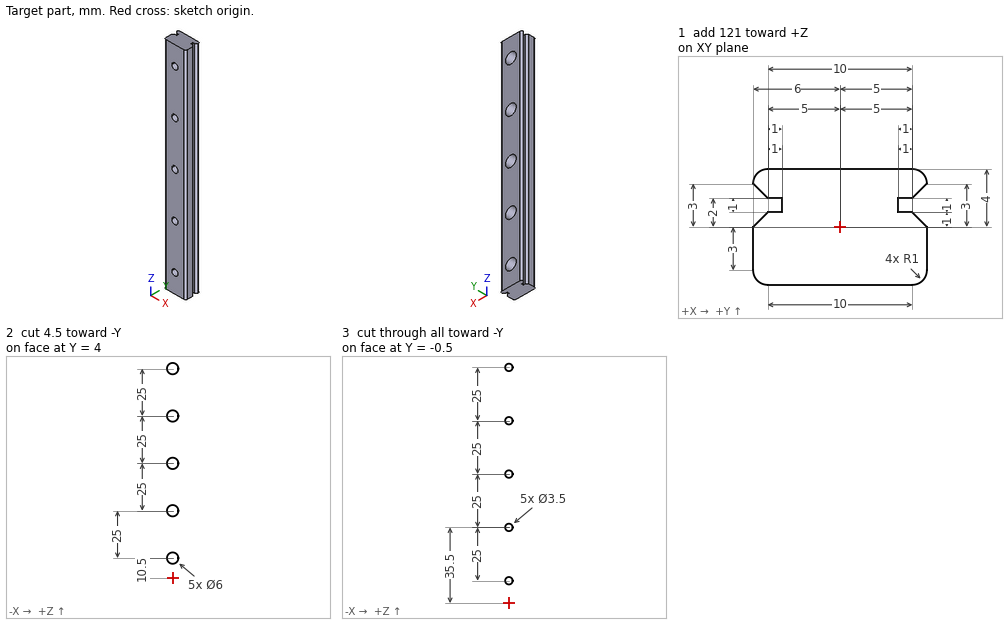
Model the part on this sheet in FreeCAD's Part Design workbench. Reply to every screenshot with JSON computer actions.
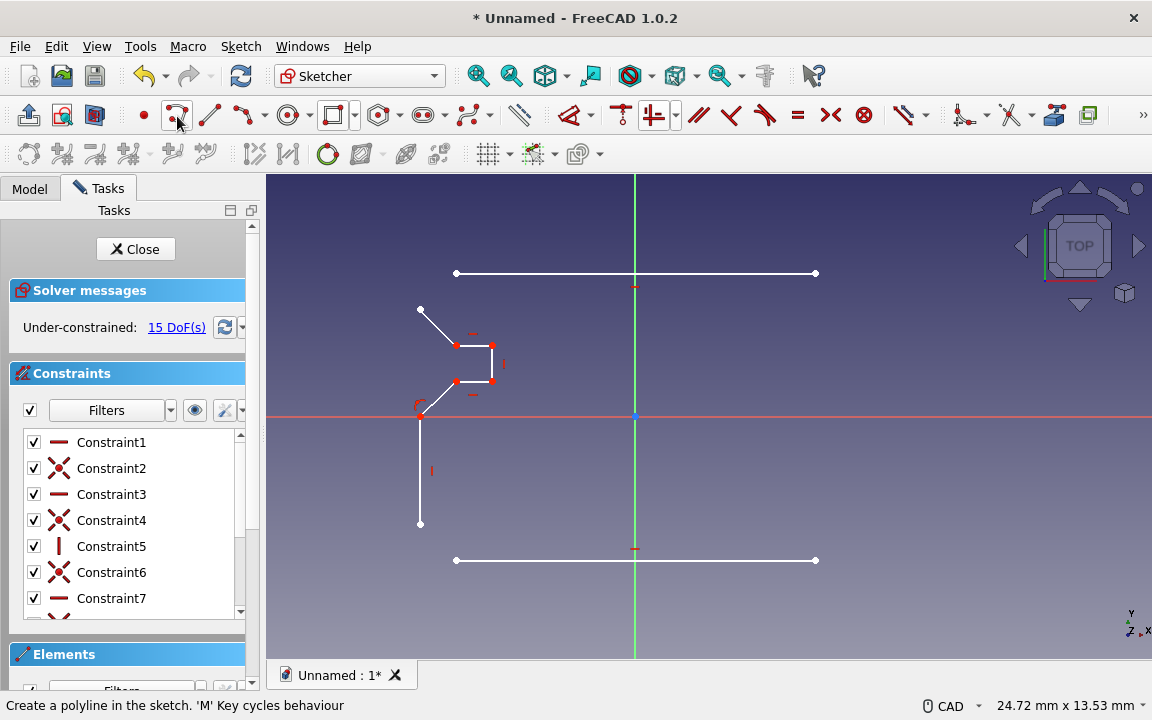
{"action": "left_click", "coordinate": [850, 524]}
{"action": "left_click", "coordinate": [850, 416]}
{"action": "left_click", "coordinate": [815, 381]}
{"action": "left_click", "coordinate": [779, 381]}
{"action": "left_click", "coordinate": [779, 345]}
{"action": "left_click", "coordinate": [815, 345]}
{"action": "left_click", "coordinate": [850, 309]}
{"action": "right_click", "coordinate": [850, 309]}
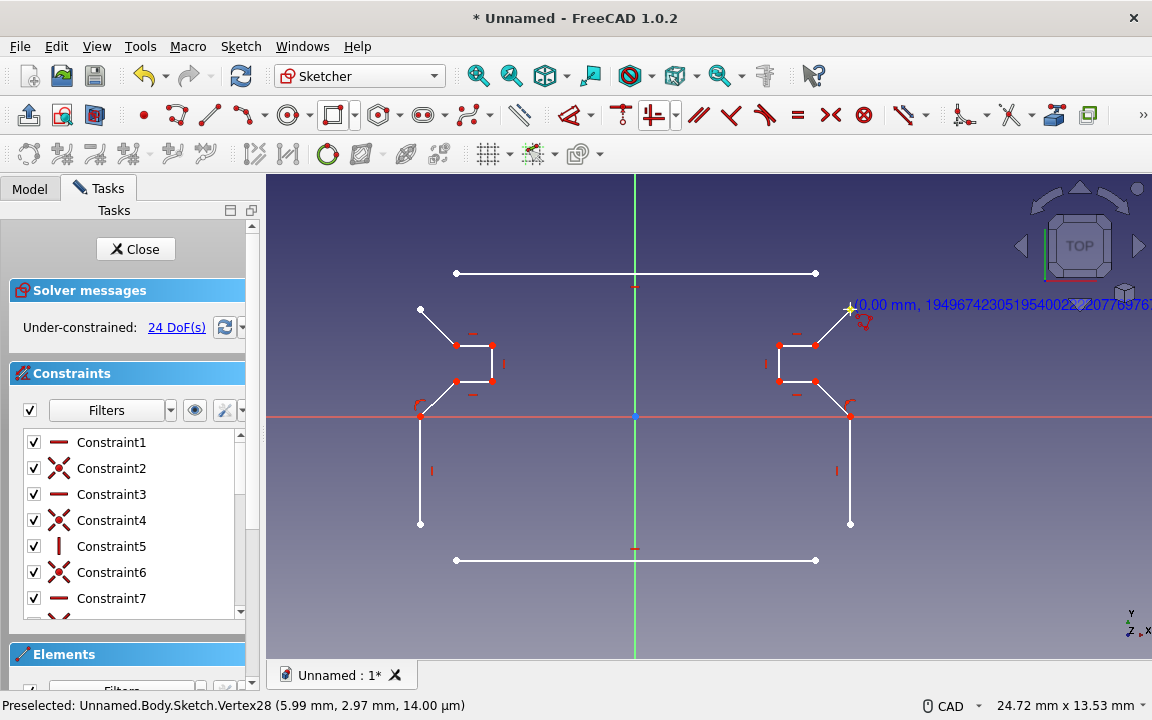
{"action": "left_click", "coordinate": [242, 116]}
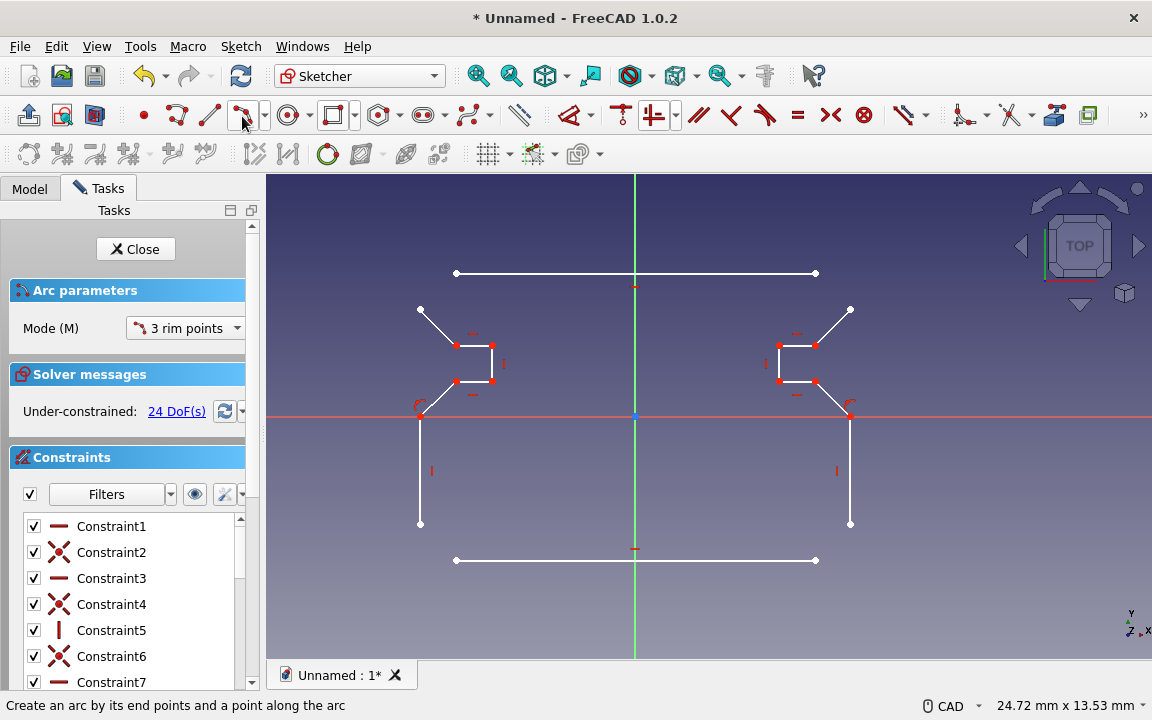
{"action": "left_click", "coordinate": [456, 274]}
{"action": "left_click", "coordinate": [420, 310]}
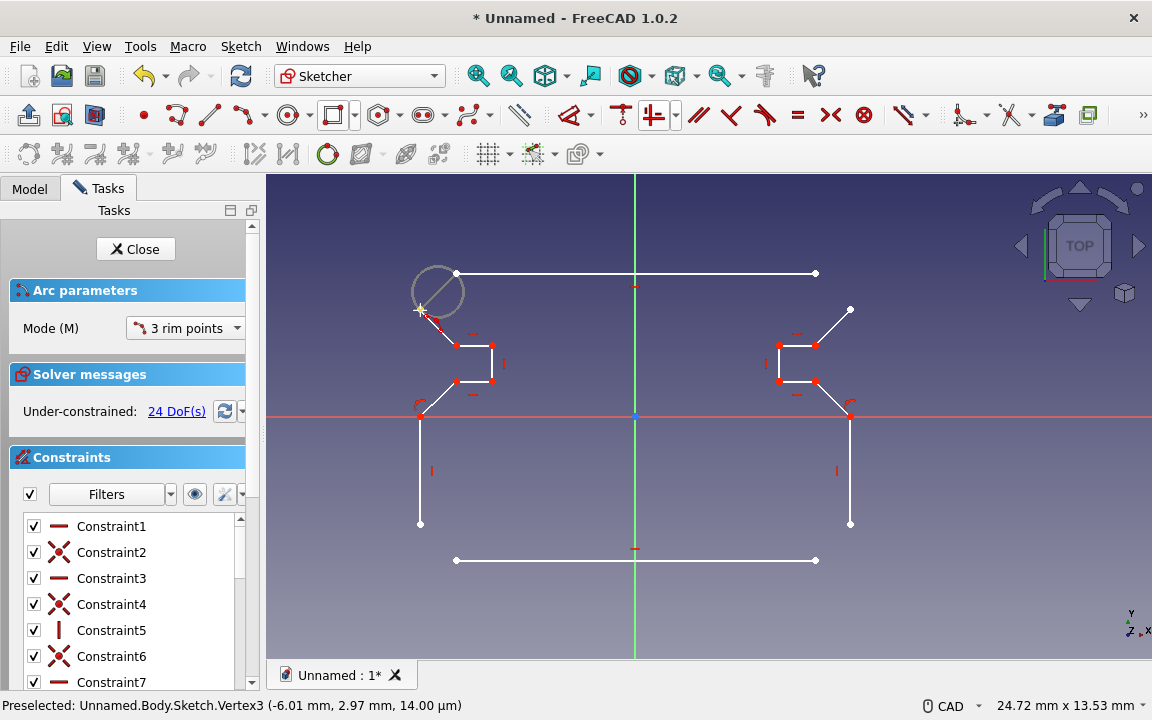
{"action": "scroll", "coordinate": [431, 284], "scroll_direction": "up", "scroll_amount": 3}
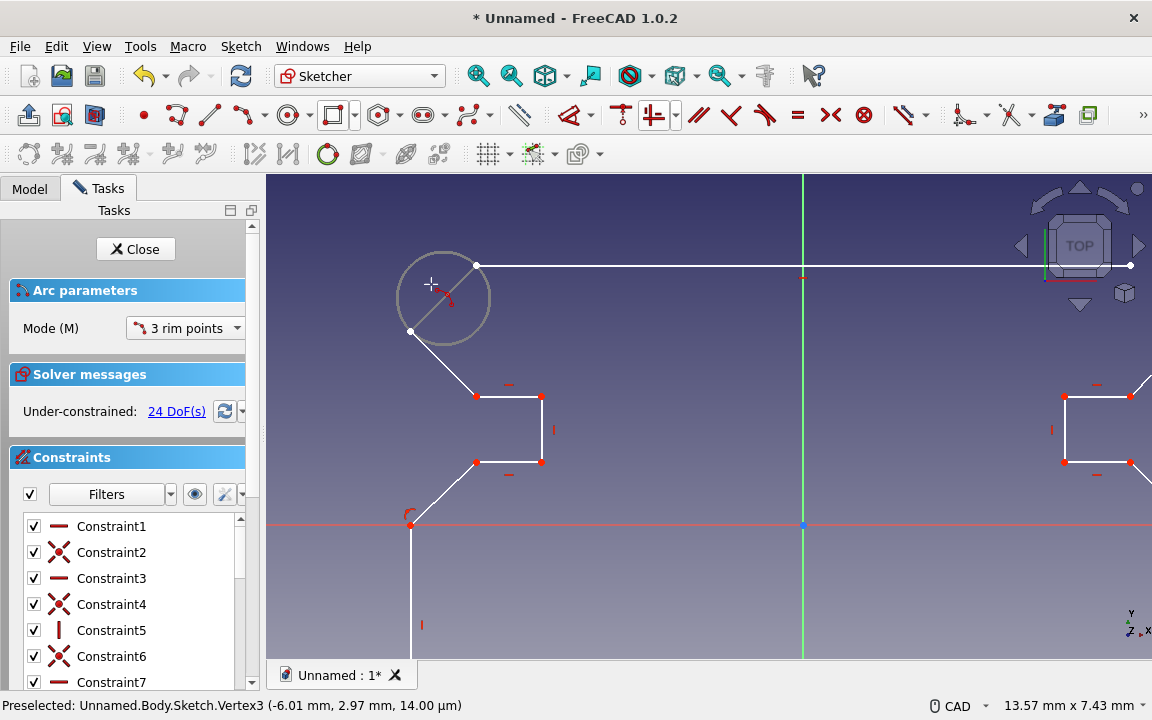
{"action": "left_click", "coordinate": [431, 283]}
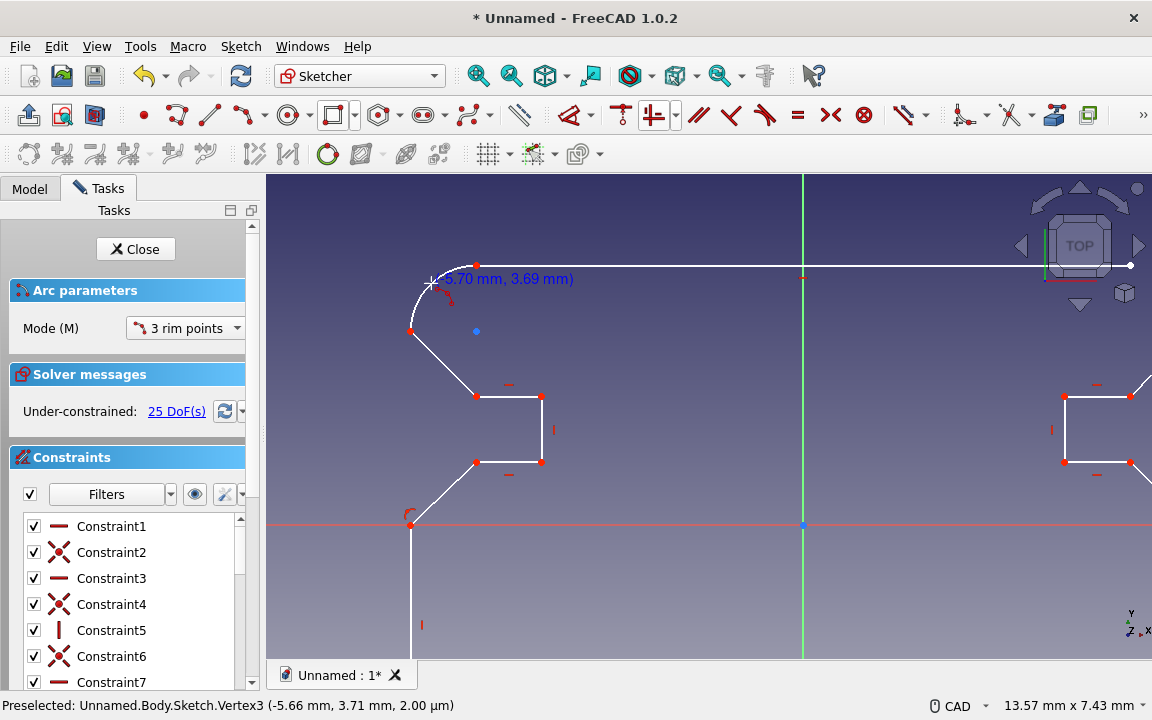
{"action": "scroll", "coordinate": [442, 284], "scroll_direction": "down", "scroll_amount": 3}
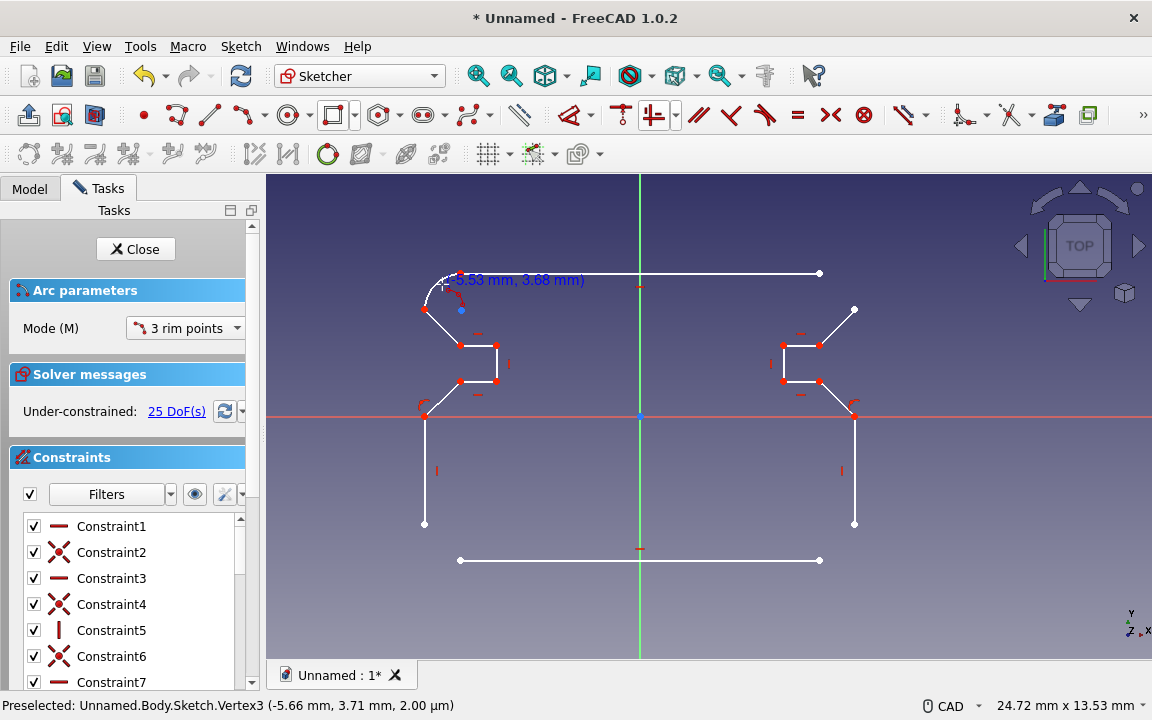
{"action": "left_click", "coordinate": [425, 525]}
{"action": "left_click", "coordinate": [461, 561]}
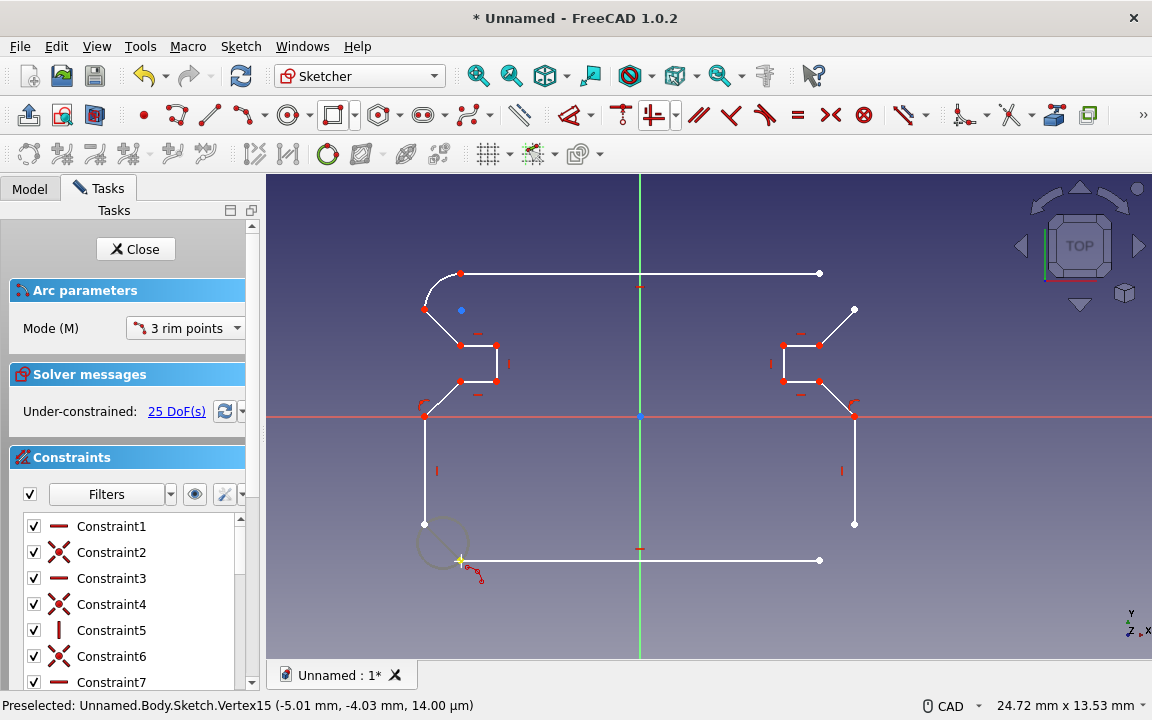
{"action": "scroll", "coordinate": [436, 549], "scroll_direction": "up", "scroll_amount": 3}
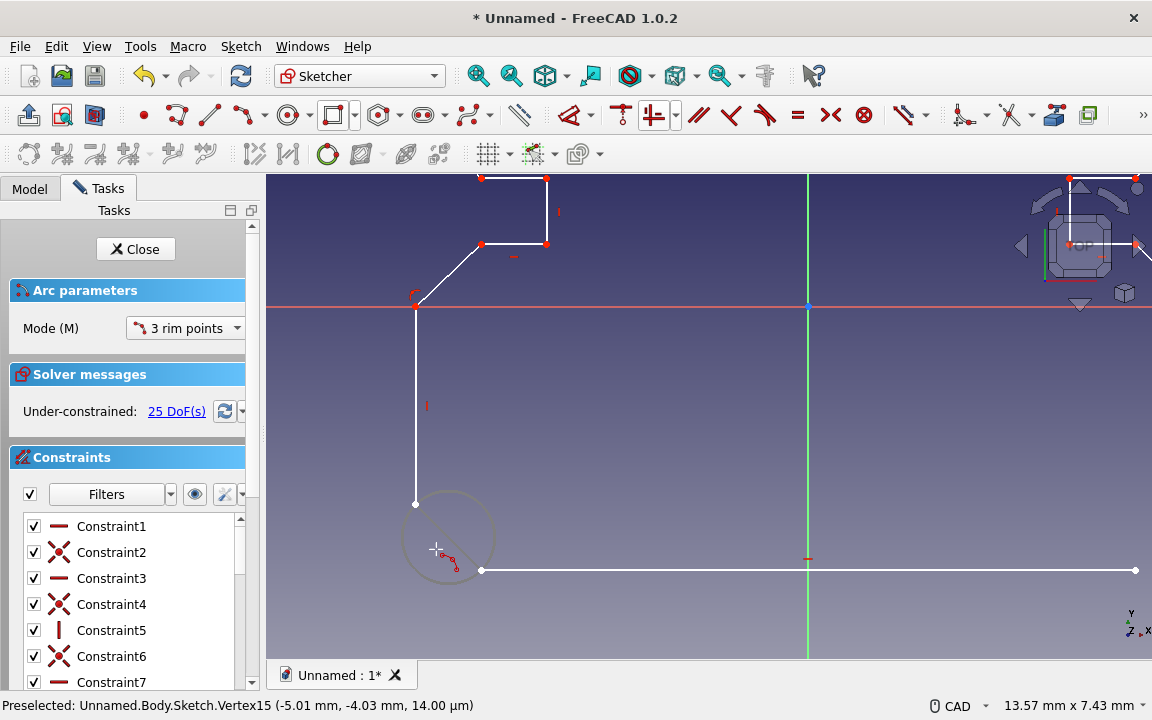
{"action": "left_click", "coordinate": [436, 549]}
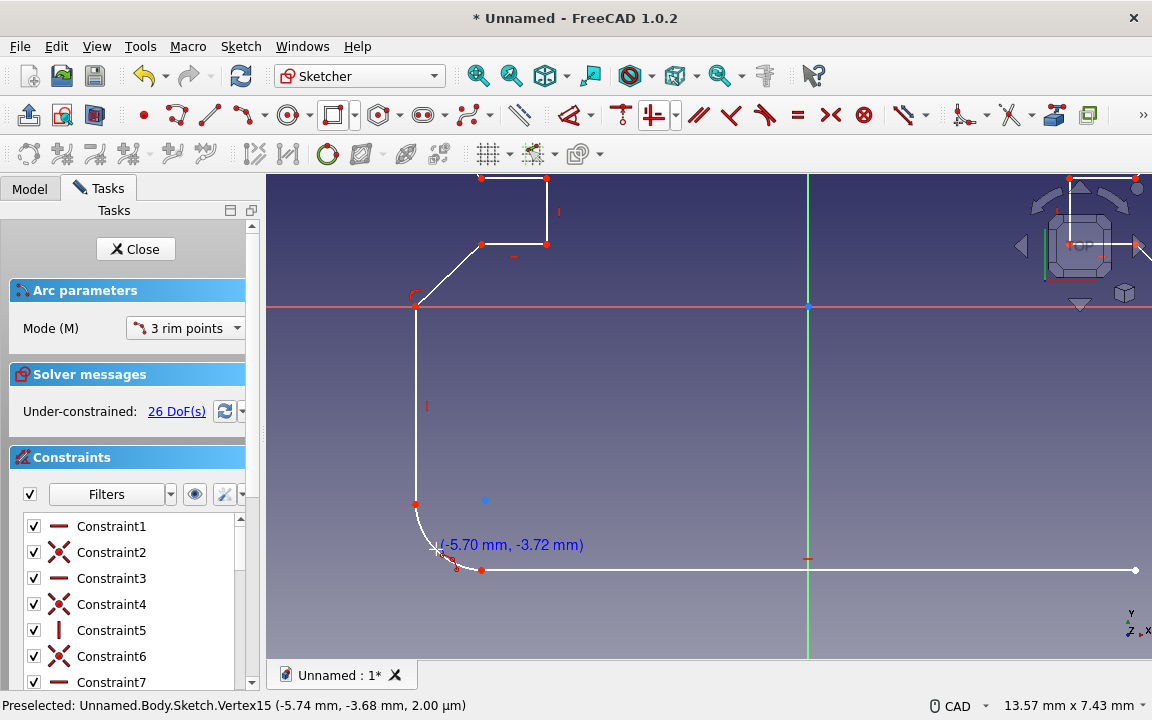
{"action": "scroll", "coordinate": [436, 550], "scroll_direction": "down", "scroll_amount": 3}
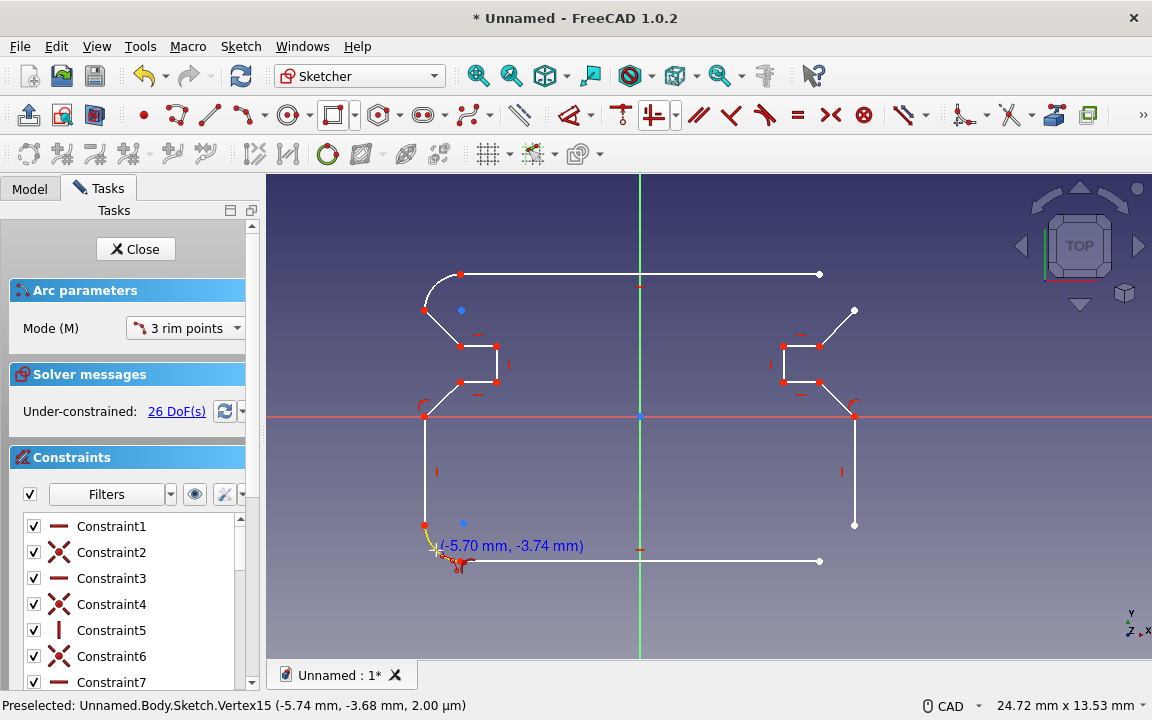
{"action": "left_click", "coordinate": [820, 561]}
{"action": "left_click", "coordinate": [855, 525]}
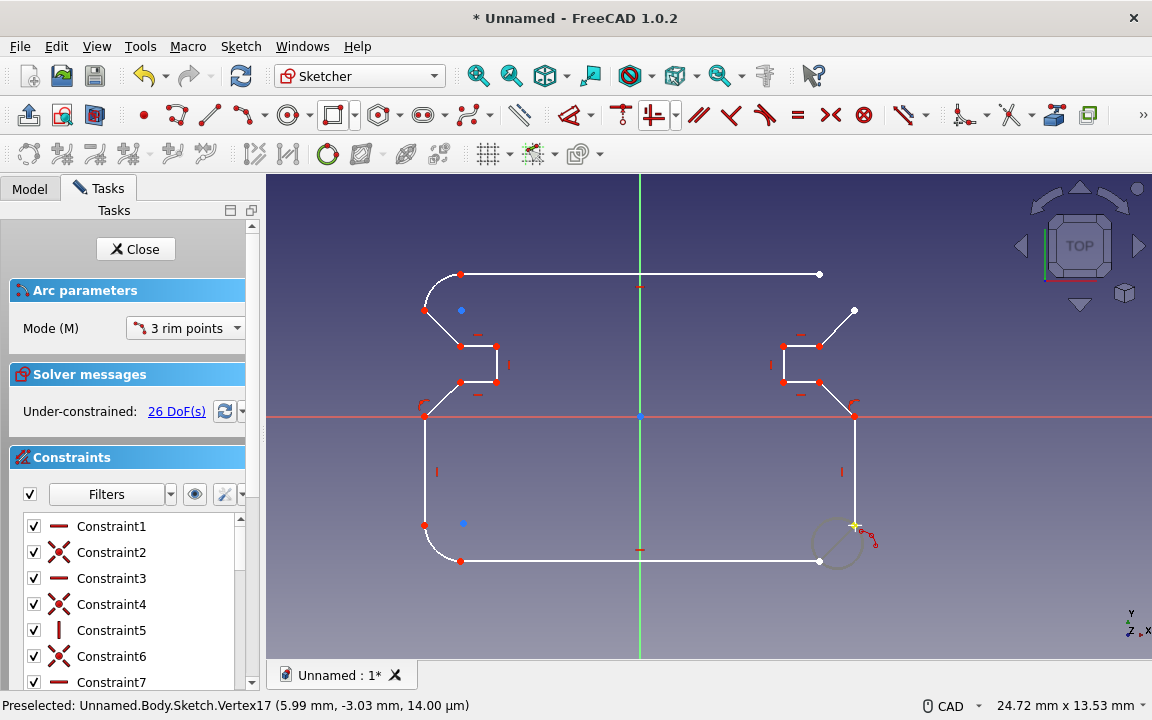
{"action": "scroll", "coordinate": [845, 550], "scroll_direction": "up", "scroll_amount": 3}